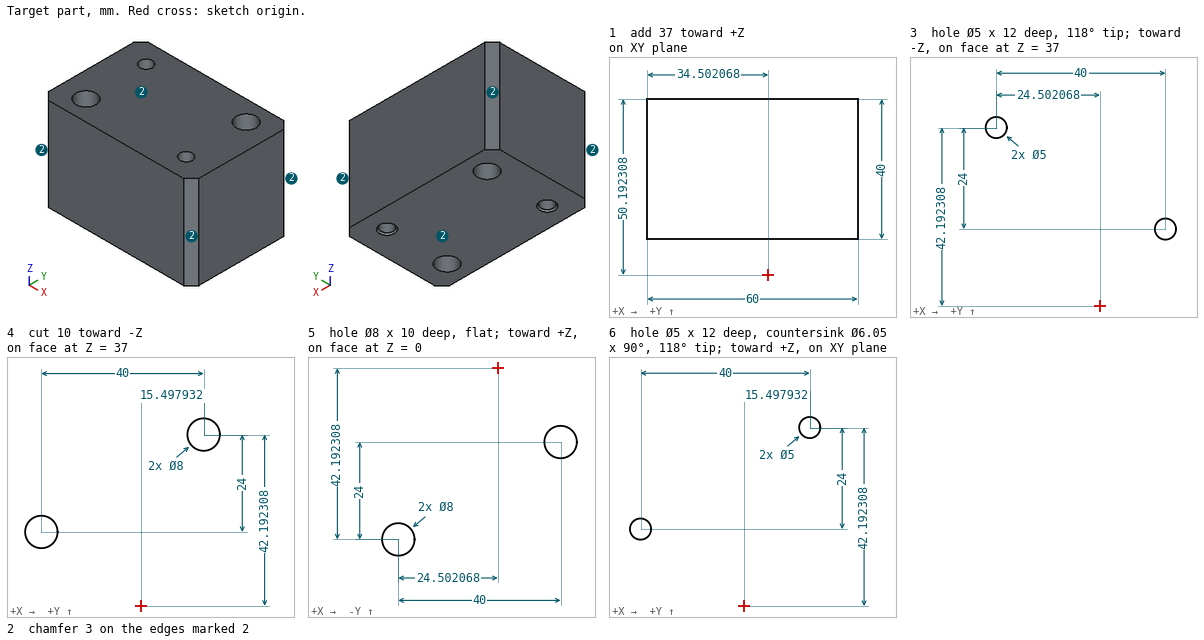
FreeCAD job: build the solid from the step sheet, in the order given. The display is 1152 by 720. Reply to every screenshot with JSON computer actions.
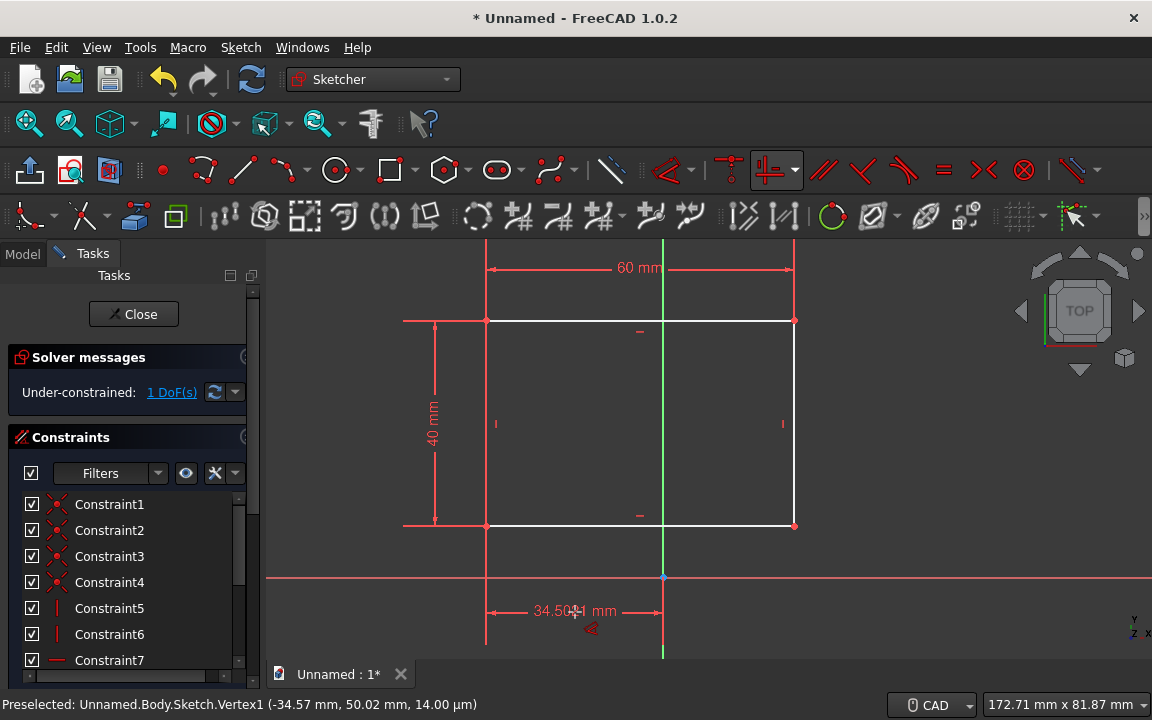
{"action": "left_click", "coordinate": [486, 321]}
{"action": "left_click", "coordinate": [452, 449]}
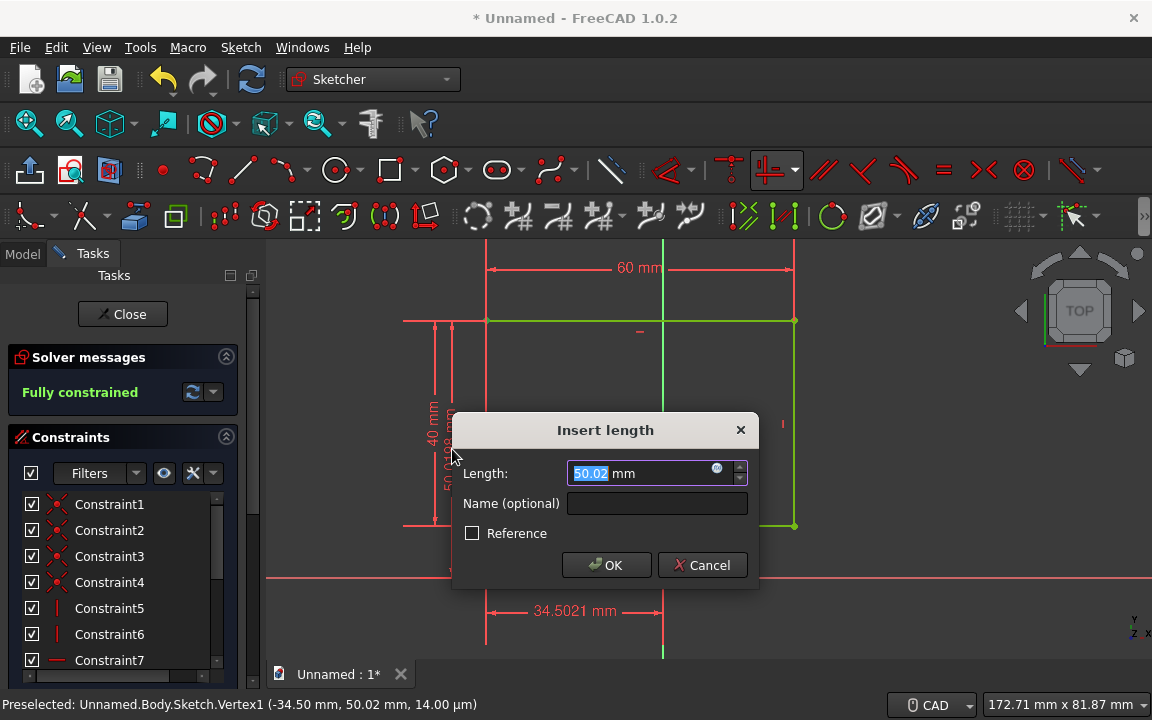
{"action": "type", "text": "50.192308"}
{"action": "key", "text": "Return"}
{"action": "key", "text": "Escape"}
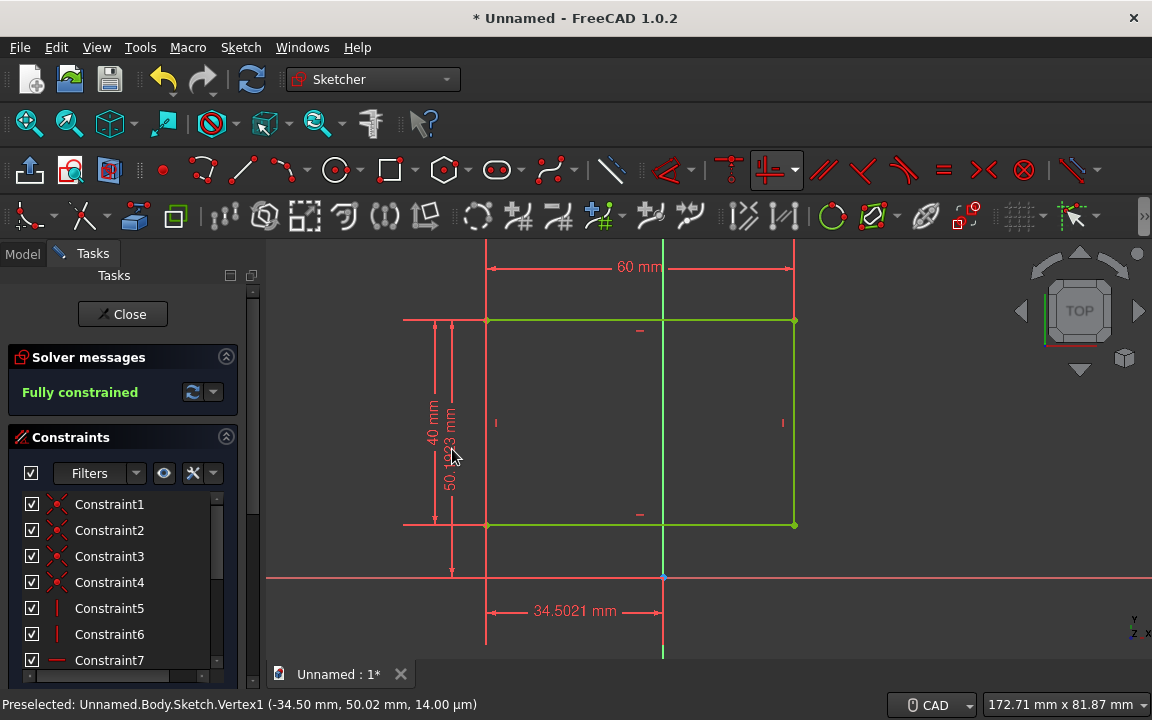
{"action": "left_click", "coordinate": [123, 314]}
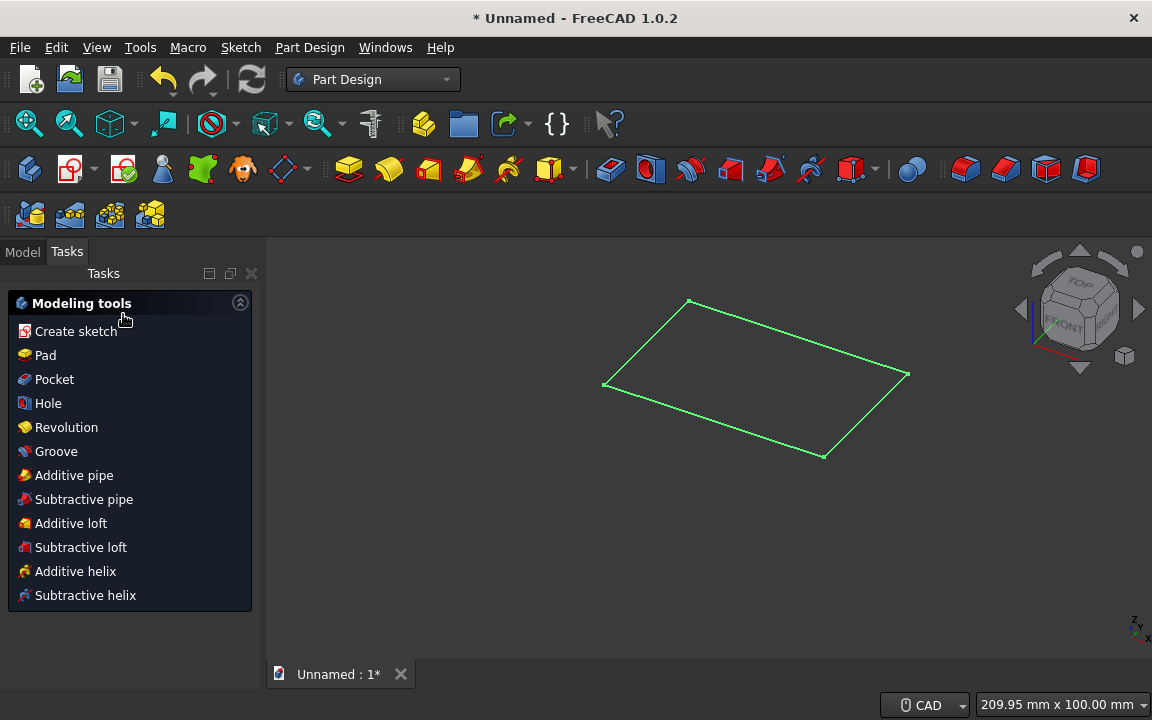
{"action": "left_click", "coordinate": [350, 170]}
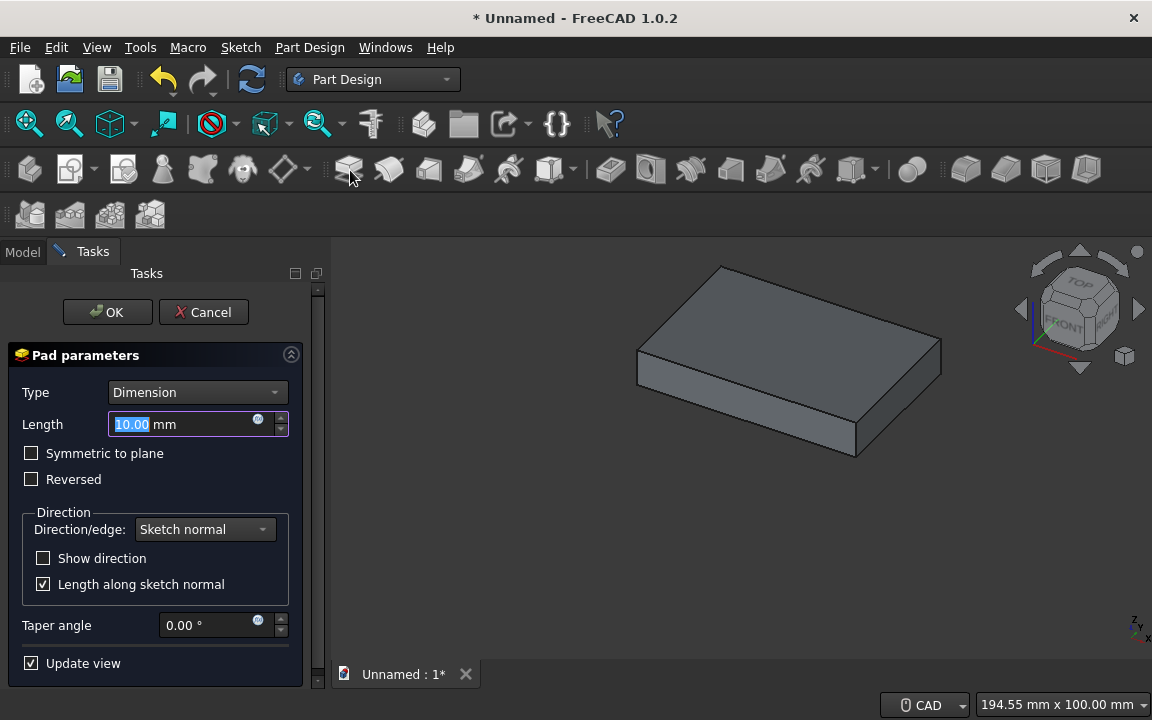
{"action": "type", "text": "37"}
{"action": "key", "text": "Tab"}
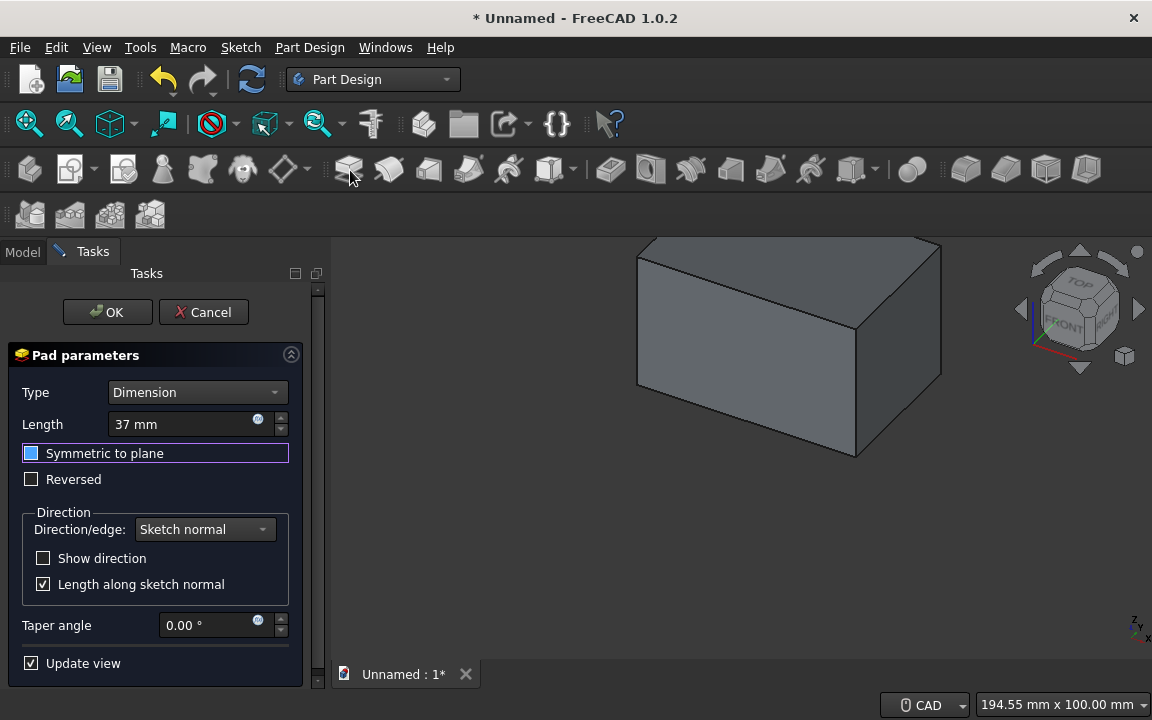
{"action": "left_click", "coordinate": [108, 312]}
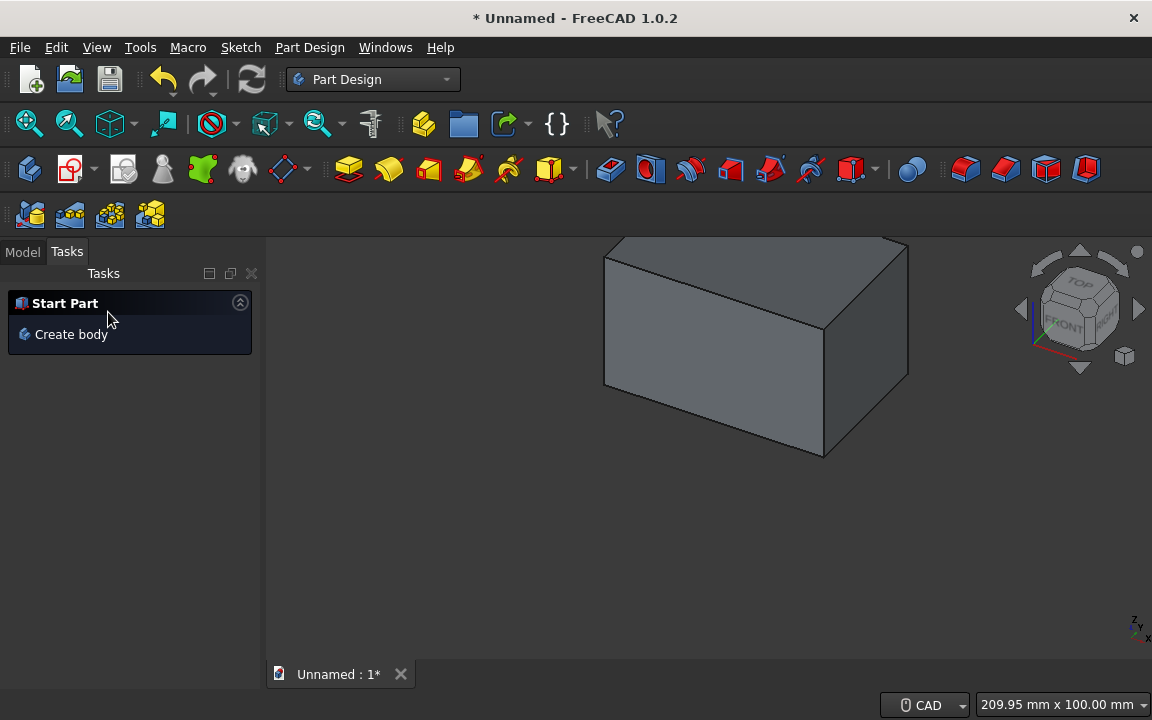
{"action": "left_click", "coordinate": [30, 124]}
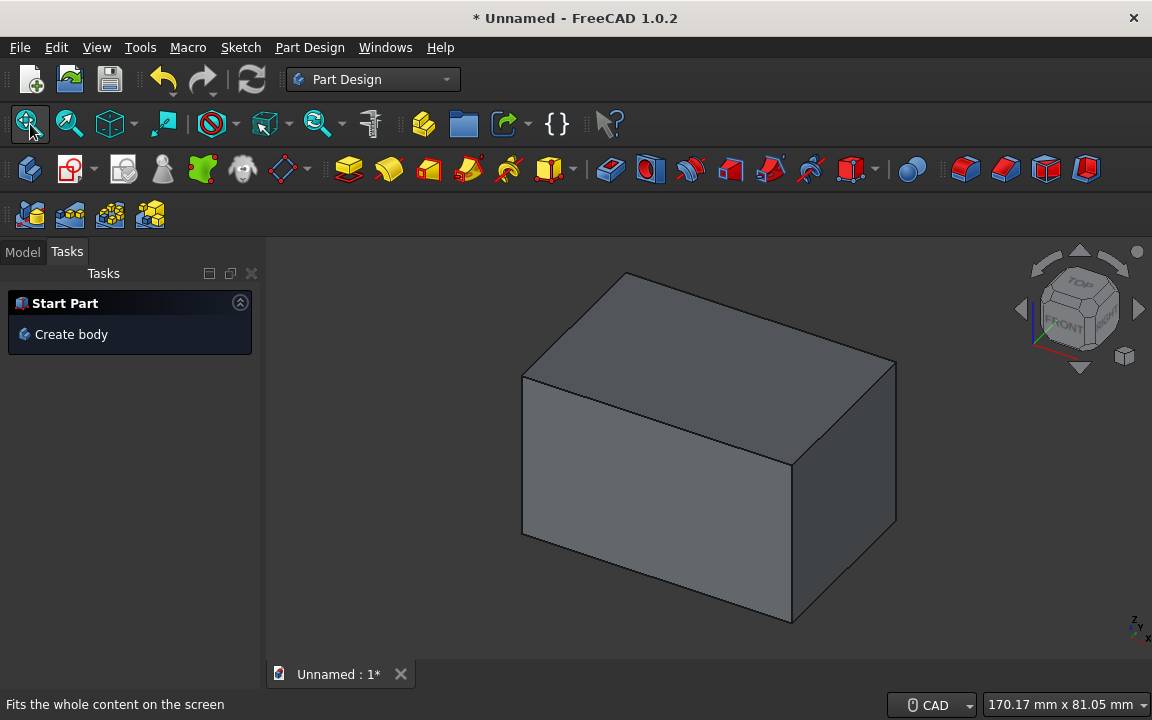
{"action": "left_click", "coordinate": [792, 544]}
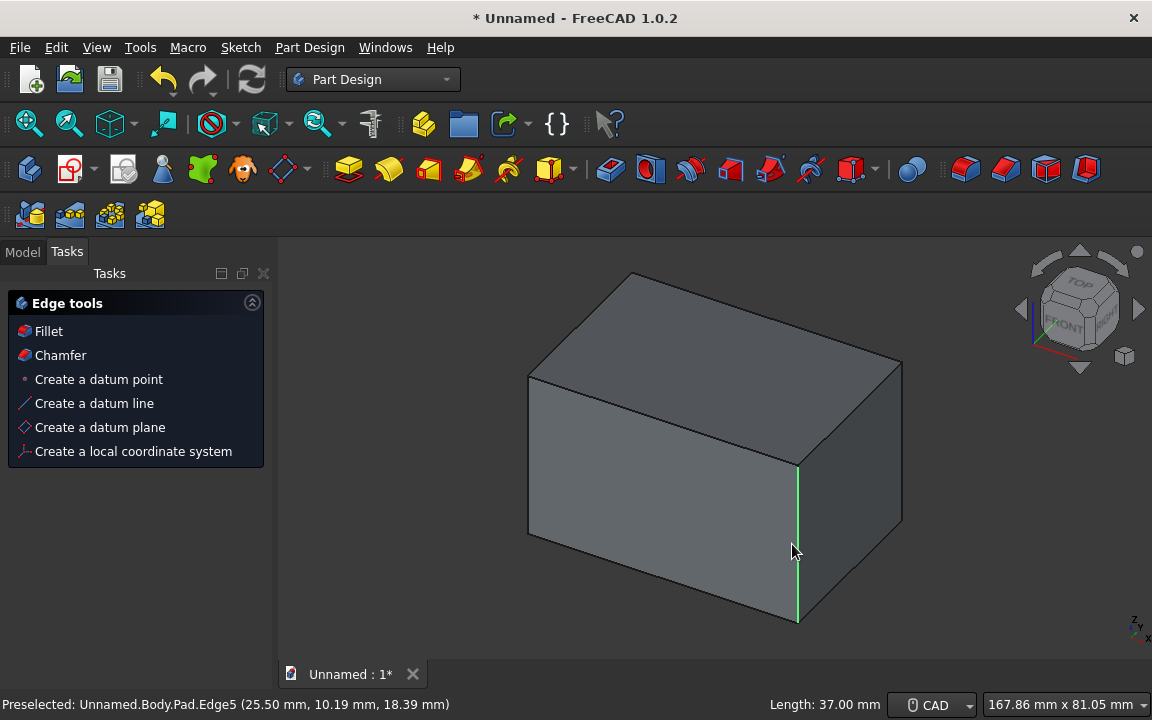
{"action": "key", "text": "0"}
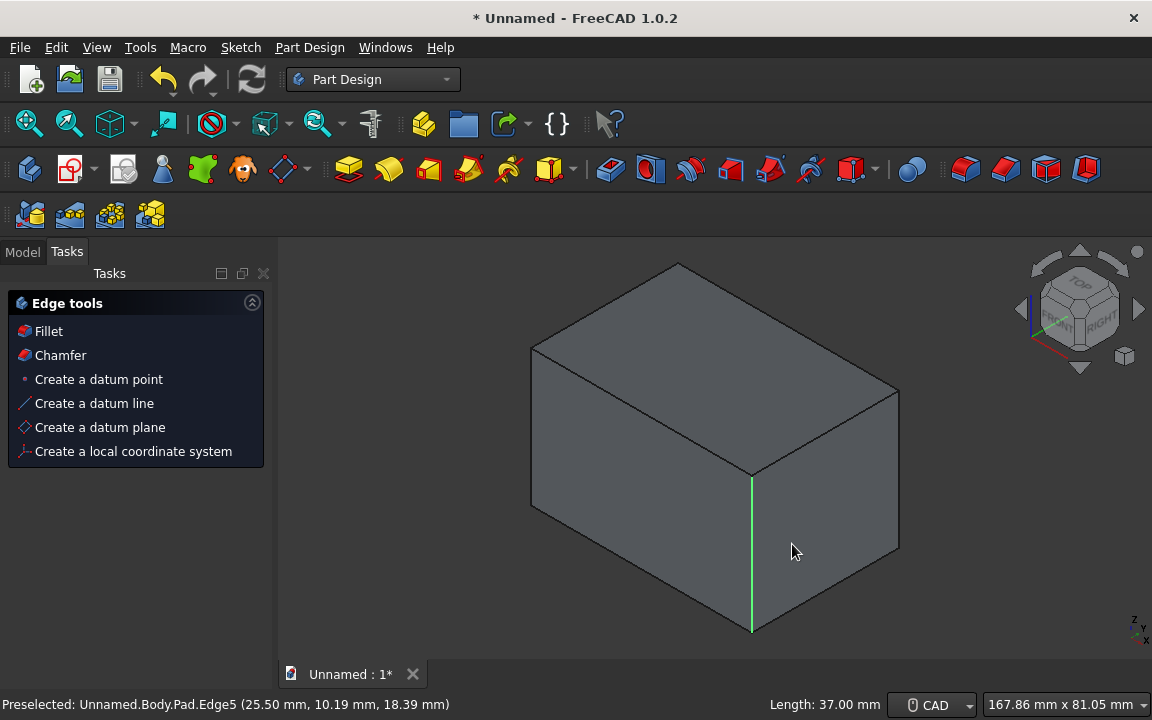
{"action": "key", "text": "2"}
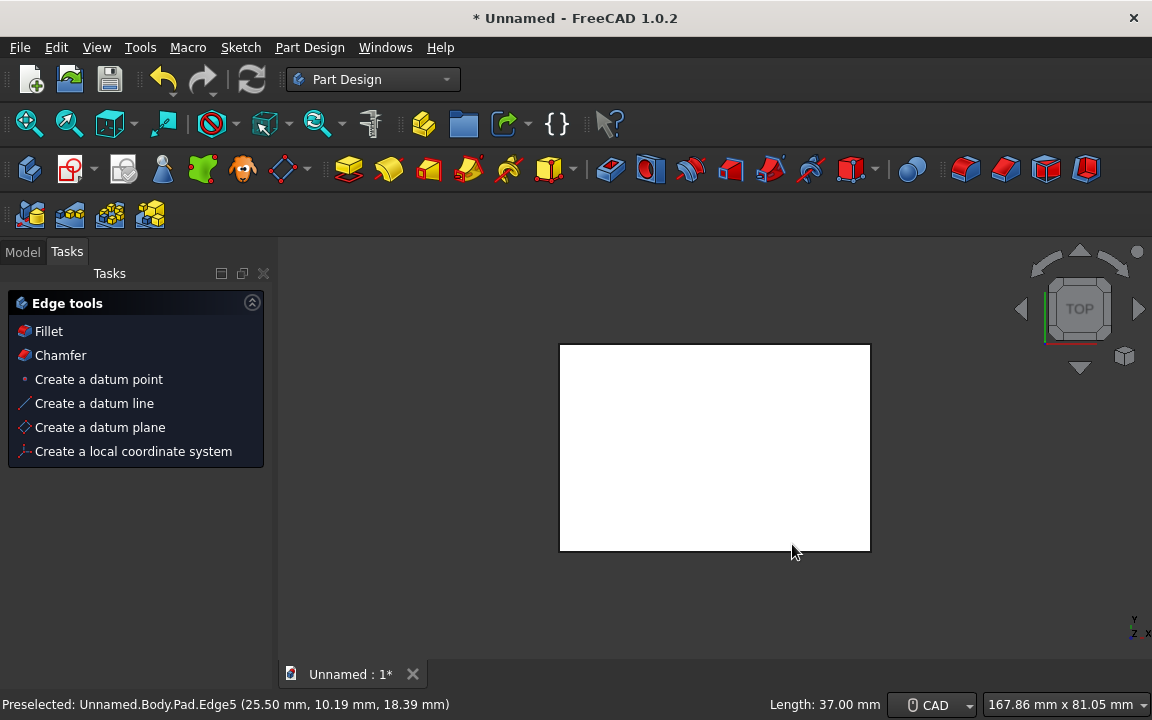
{"action": "key", "text": "1"}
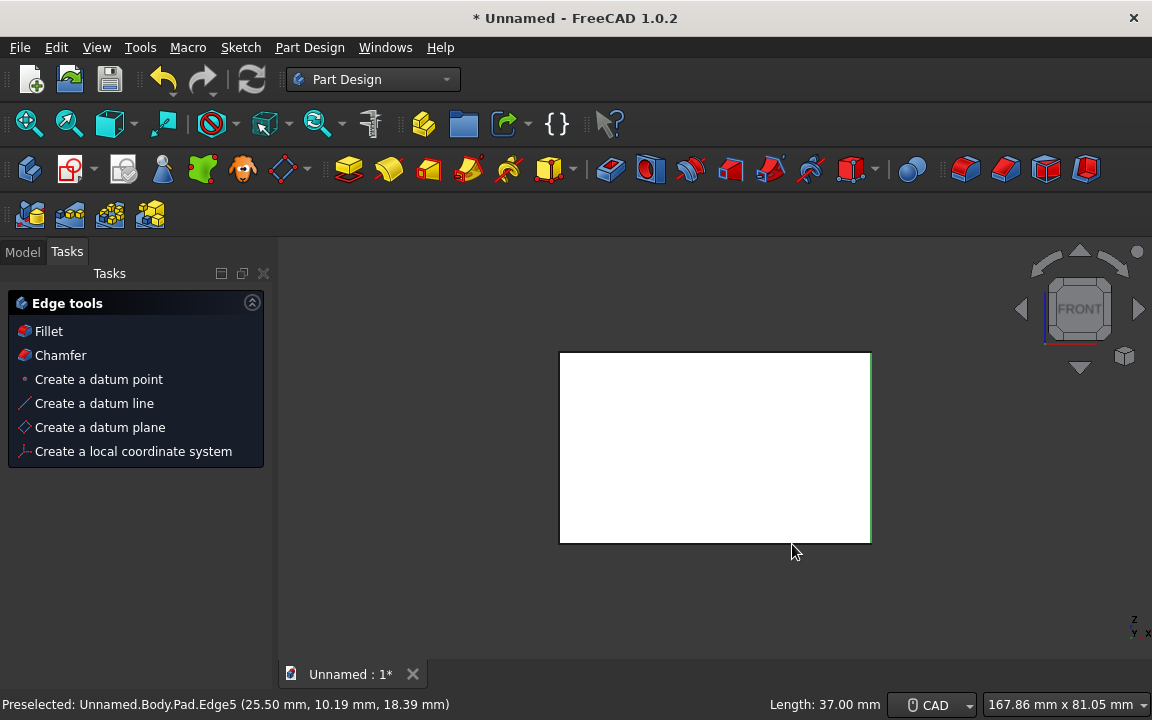
{"action": "left_click", "coordinate": [559, 447], "text": "ctrl"}